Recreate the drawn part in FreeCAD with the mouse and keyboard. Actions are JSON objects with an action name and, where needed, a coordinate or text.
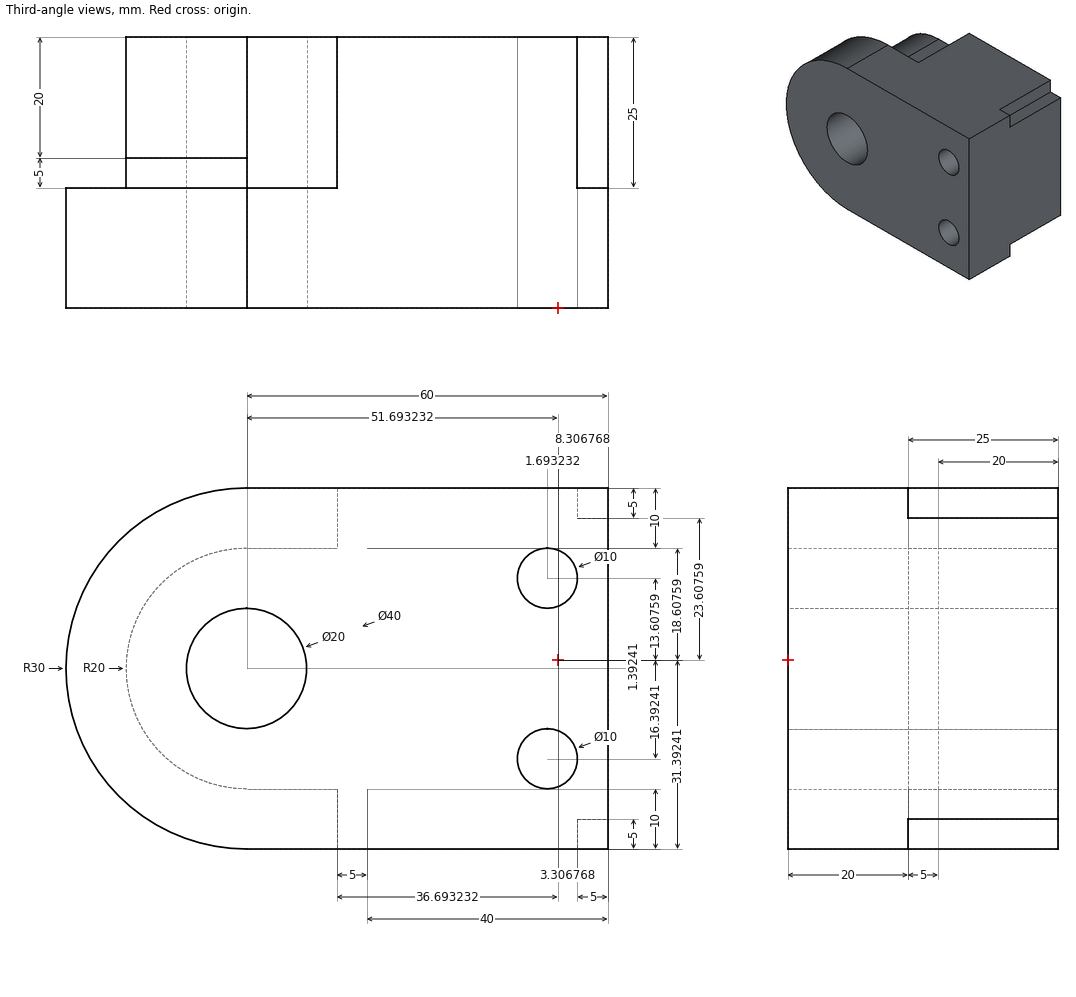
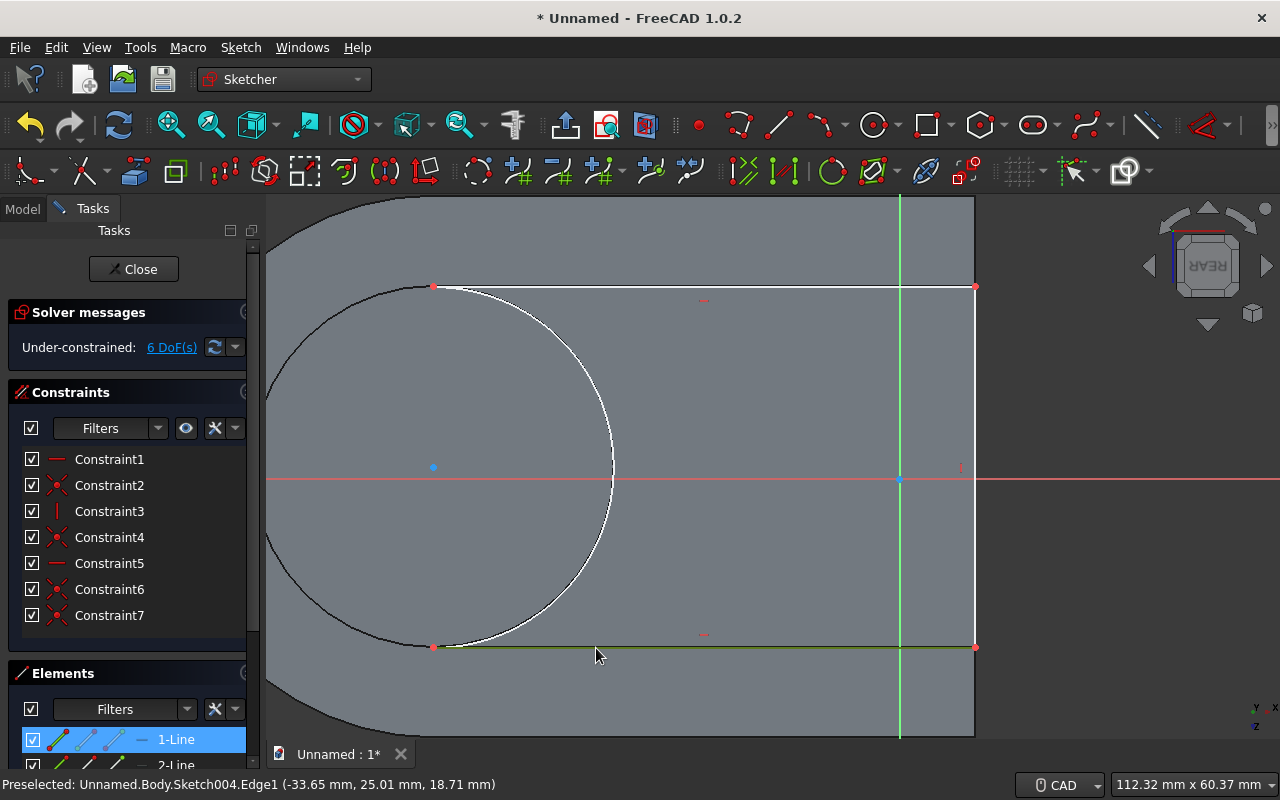
{"action": "left_click", "coordinate": [579, 574]}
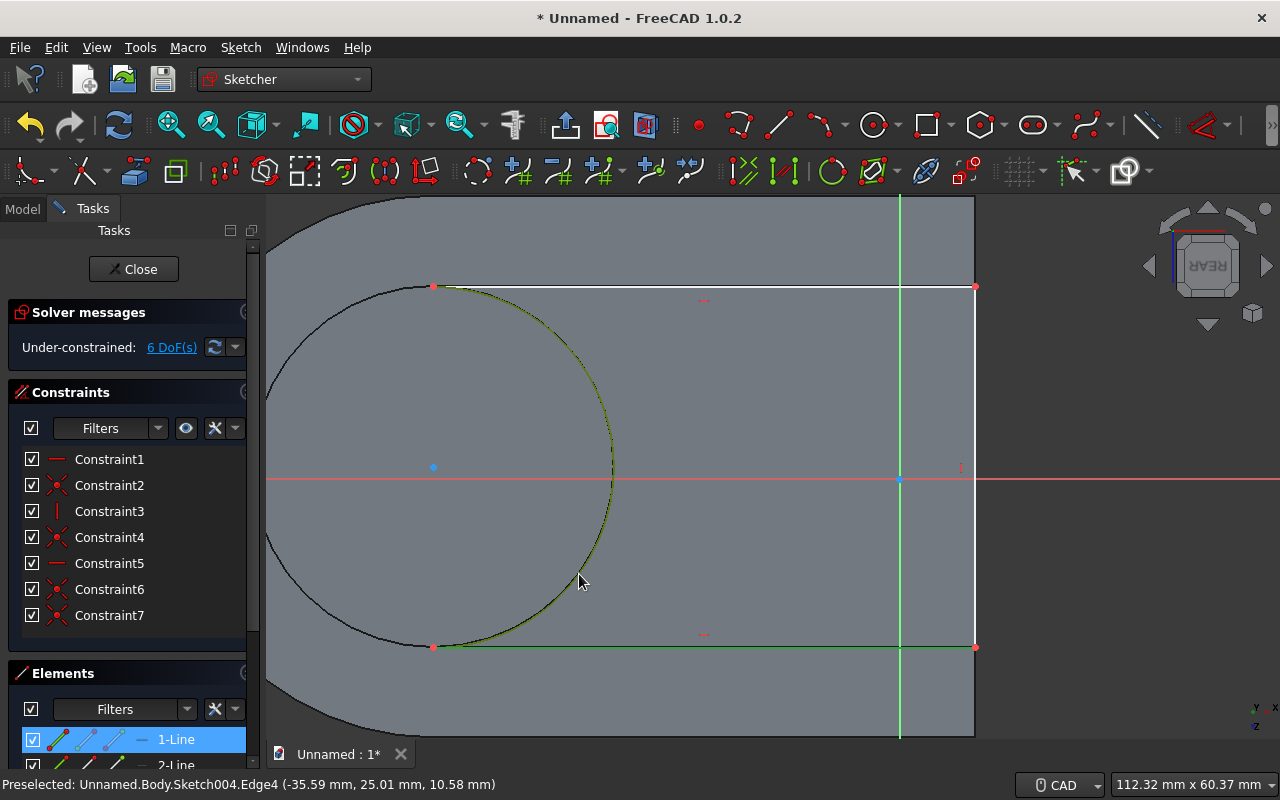
{"action": "key", "text": "t"}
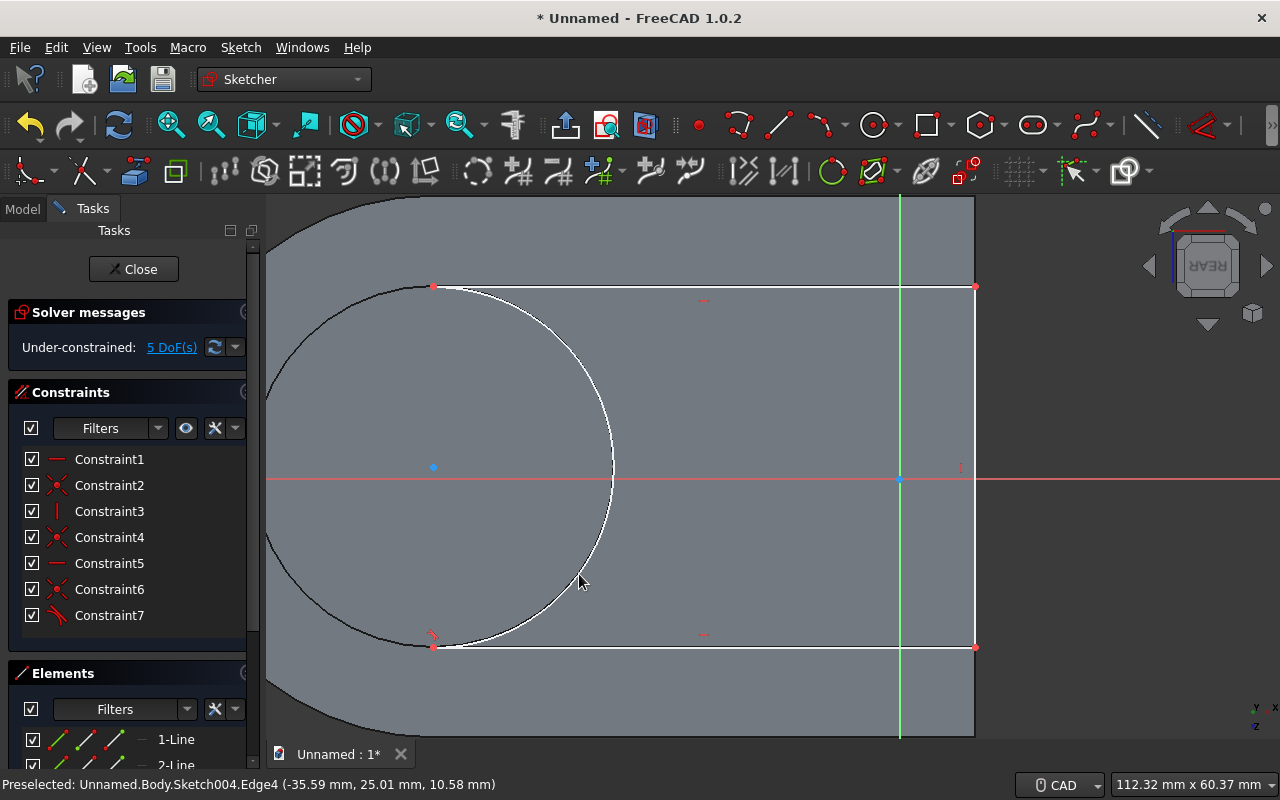
{"action": "left_click", "coordinate": [812, 287]}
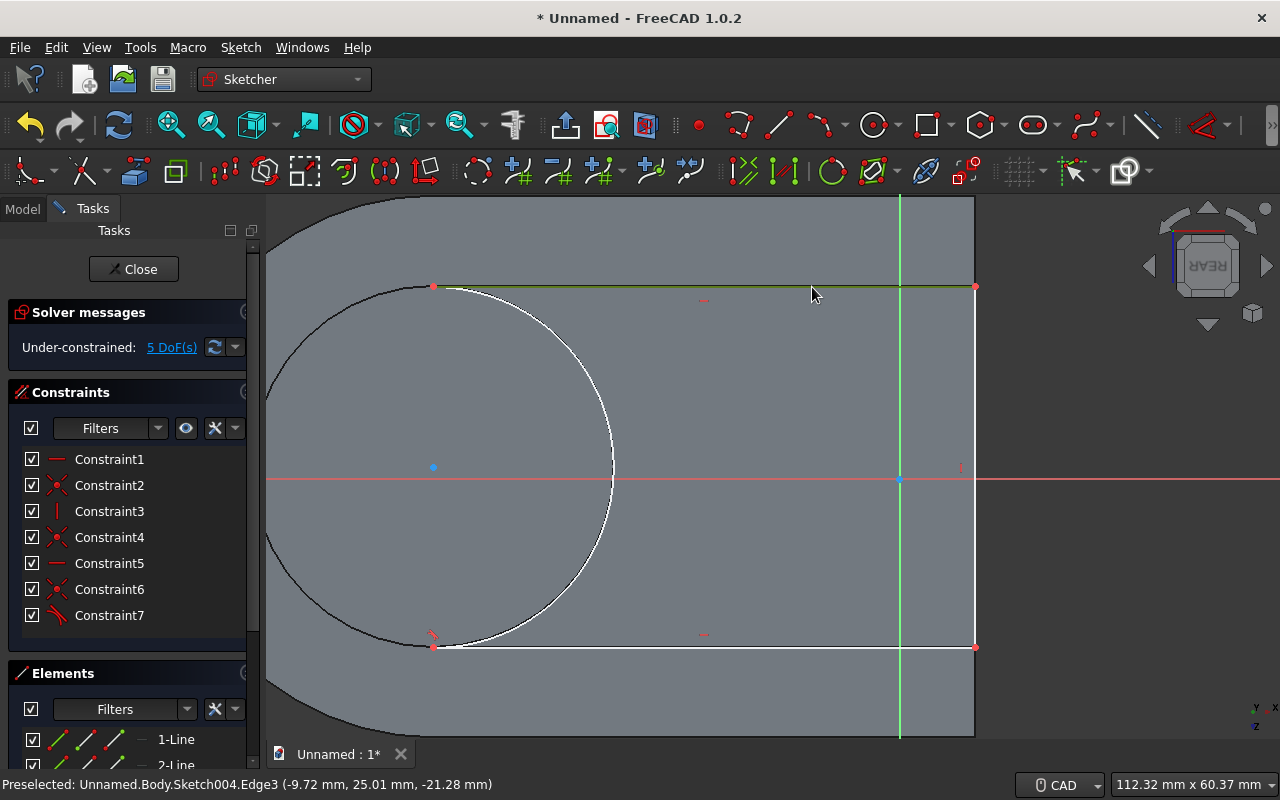
{"action": "left_click", "coordinate": [579, 574]}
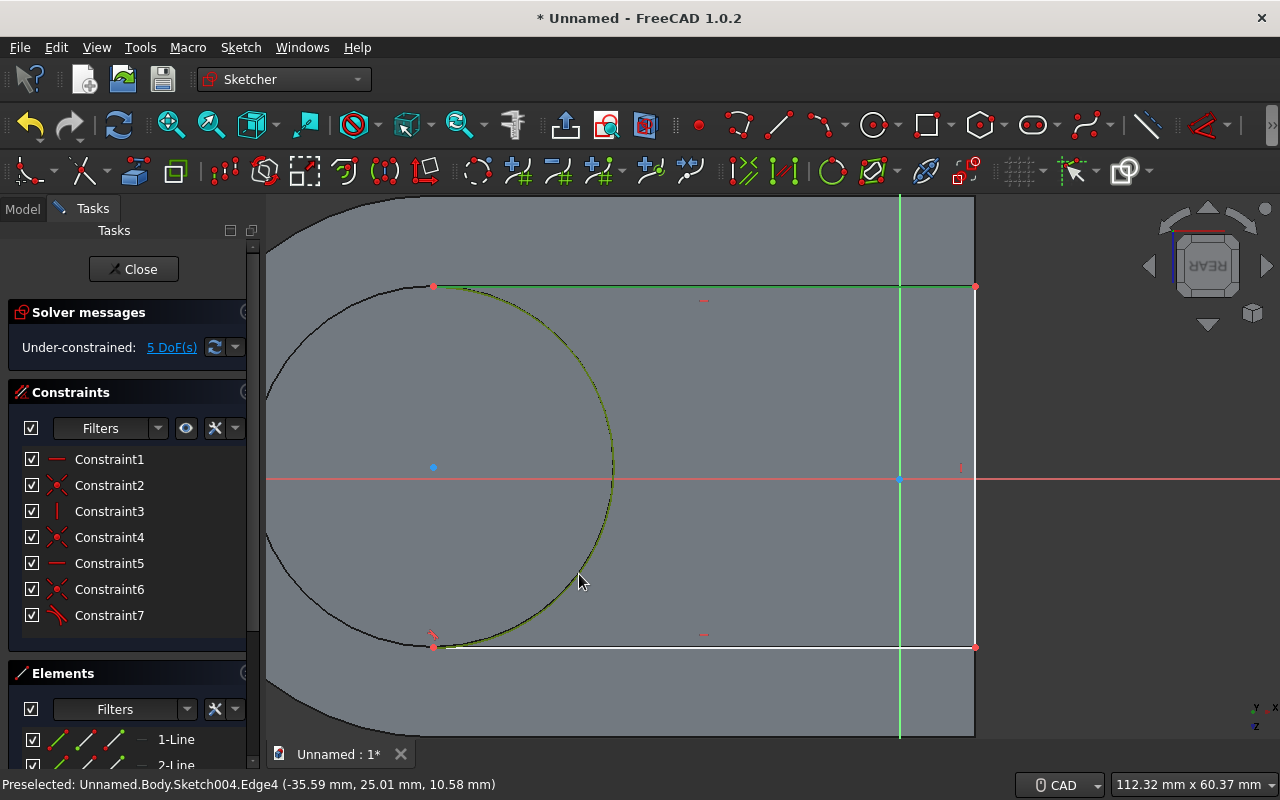
{"action": "key", "text": "t"}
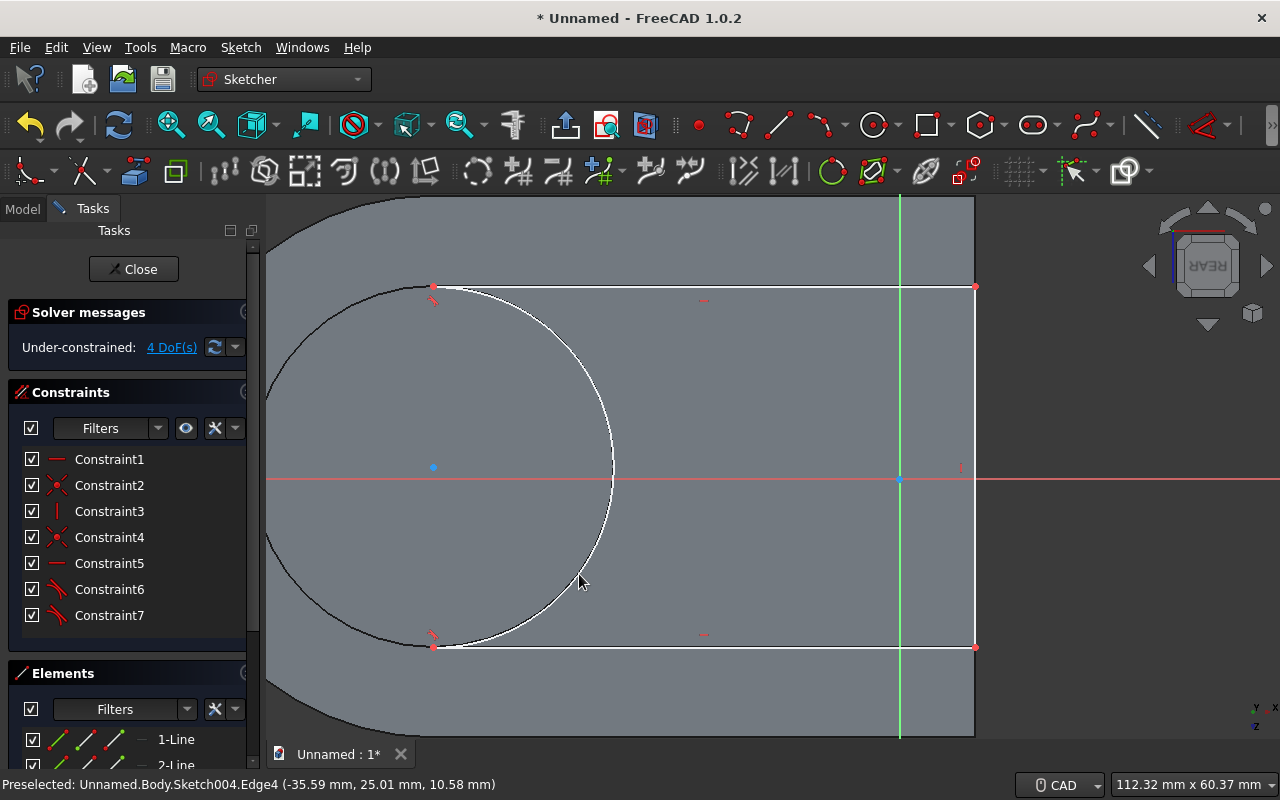
{"action": "key", "text": "d"}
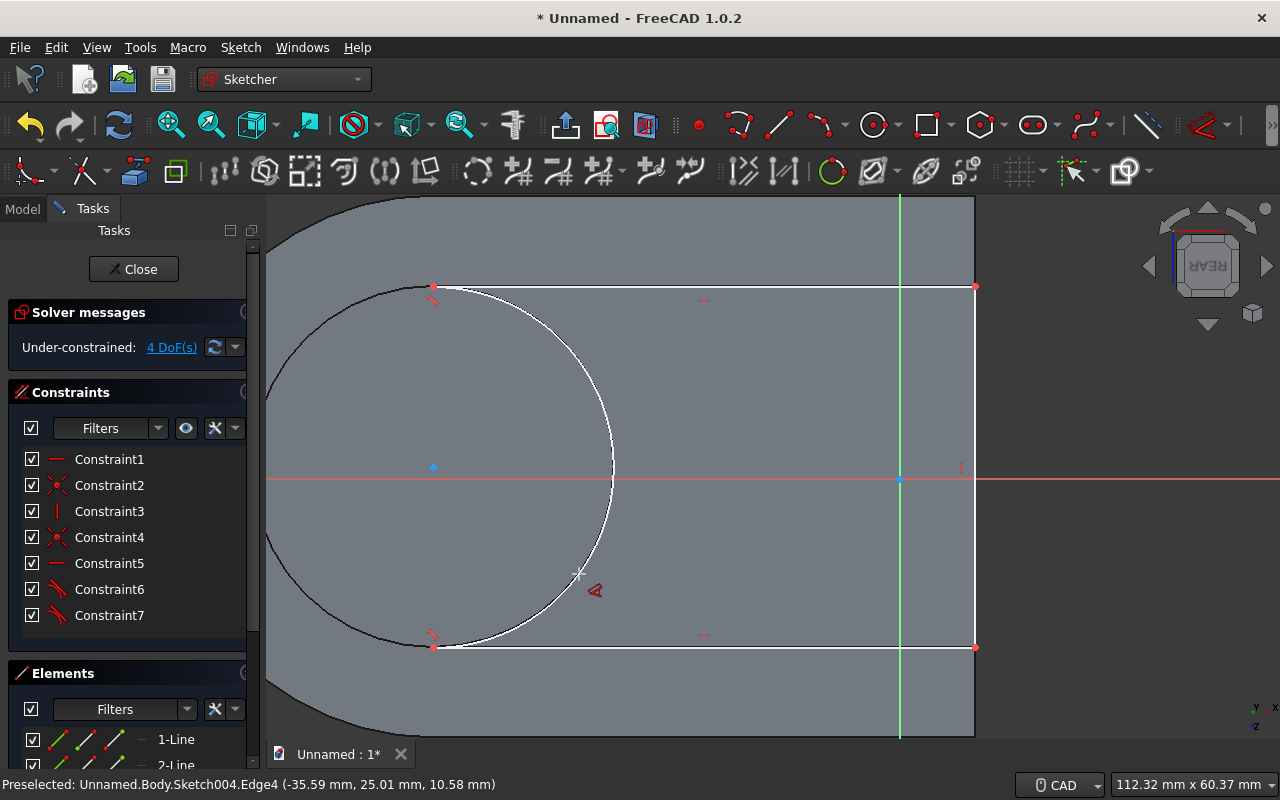
{"action": "left_click", "coordinate": [579, 574]}
{"action": "left_click", "coordinate": [605, 593]}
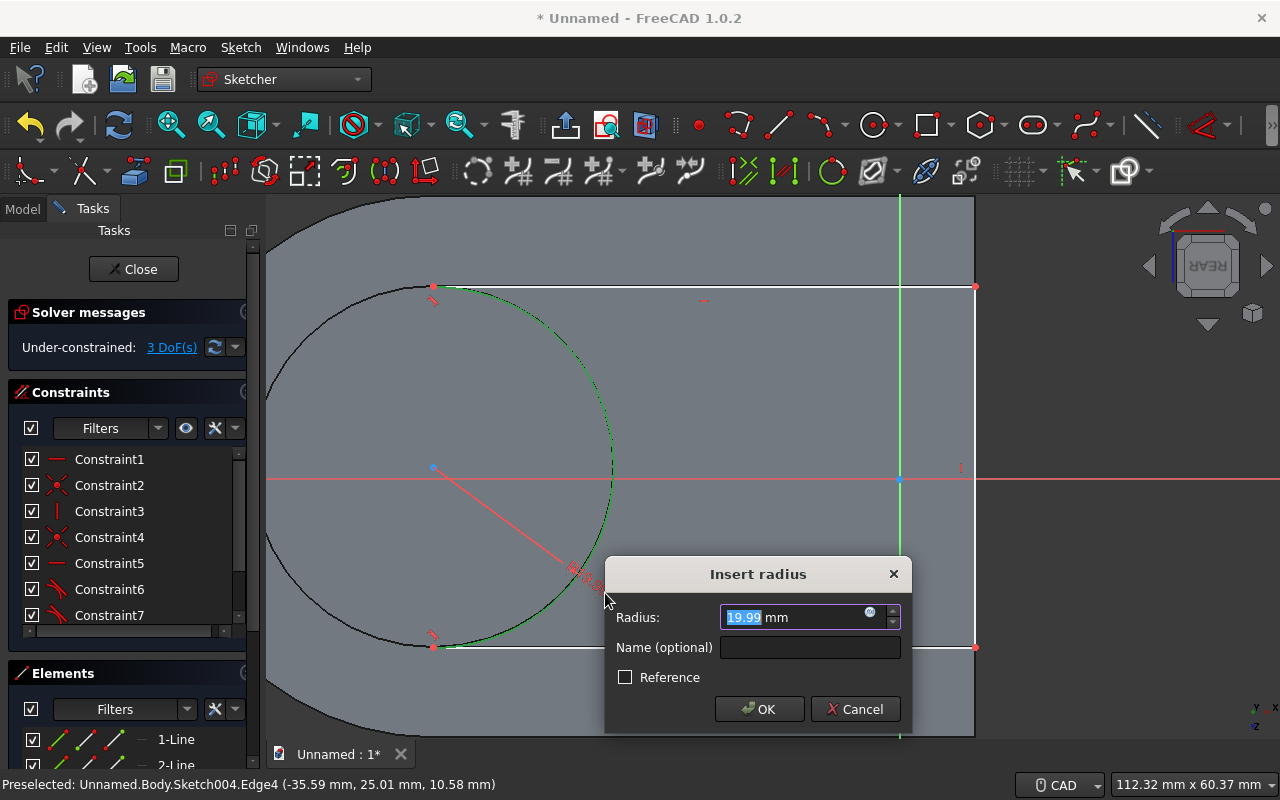
{"action": "type", "text": "20"}
{"action": "key", "text": "Return"}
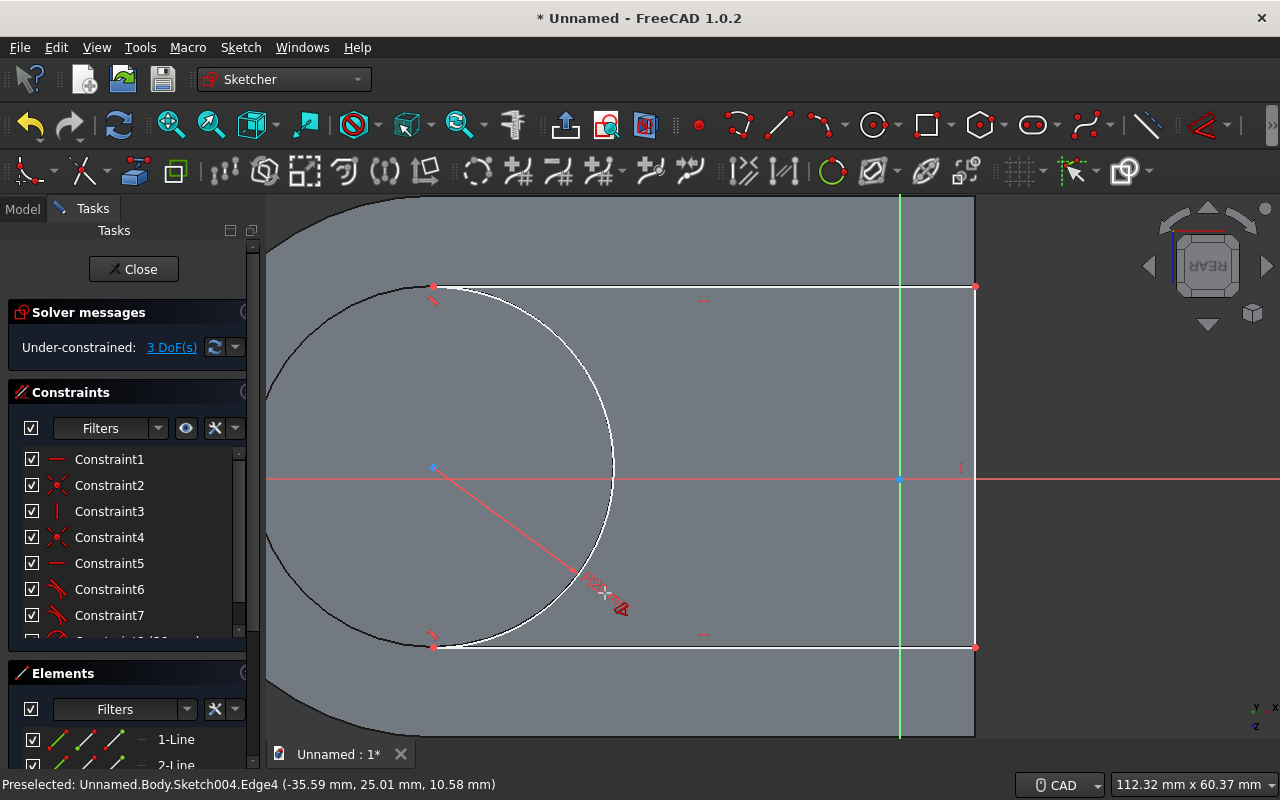
{"action": "left_click", "coordinate": [596, 648]}
{"action": "left_click", "coordinate": [704, 682]}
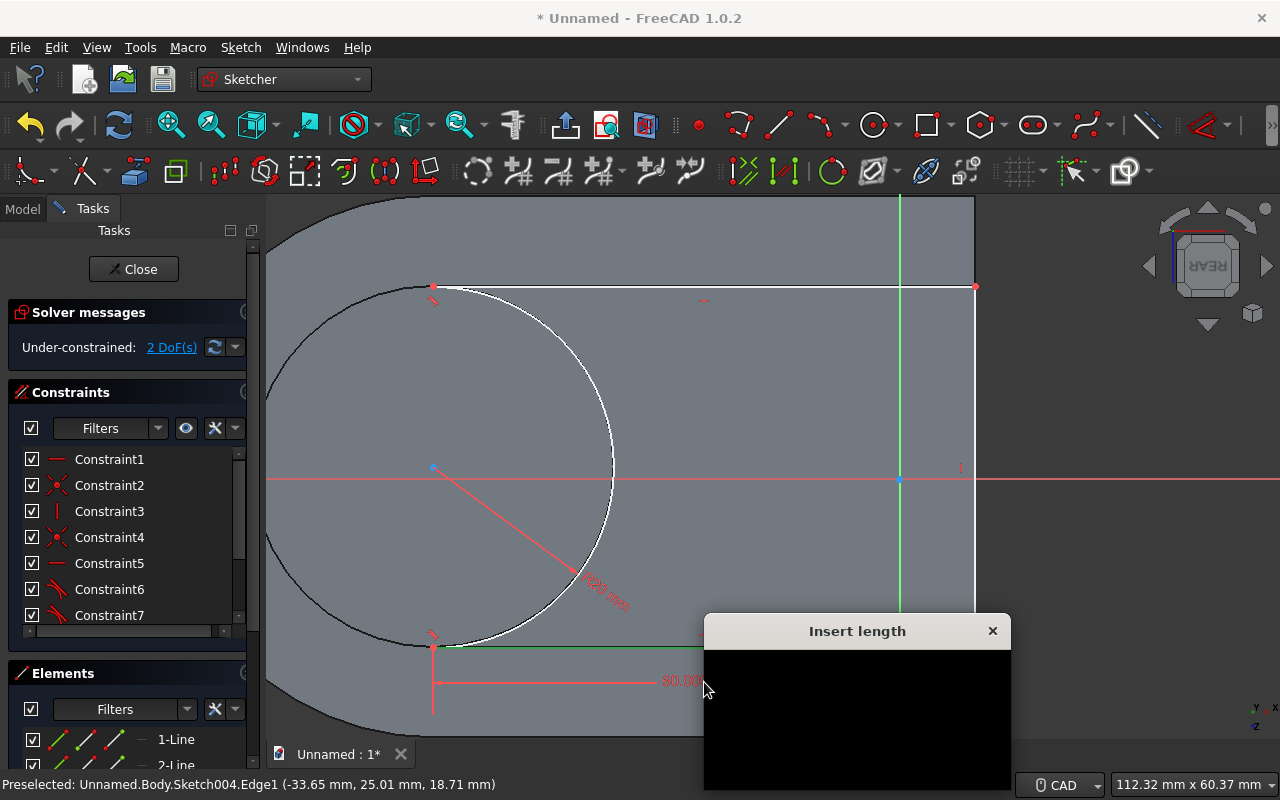
{"action": "type", "text": "60"}
{"action": "key", "text": "Return"}